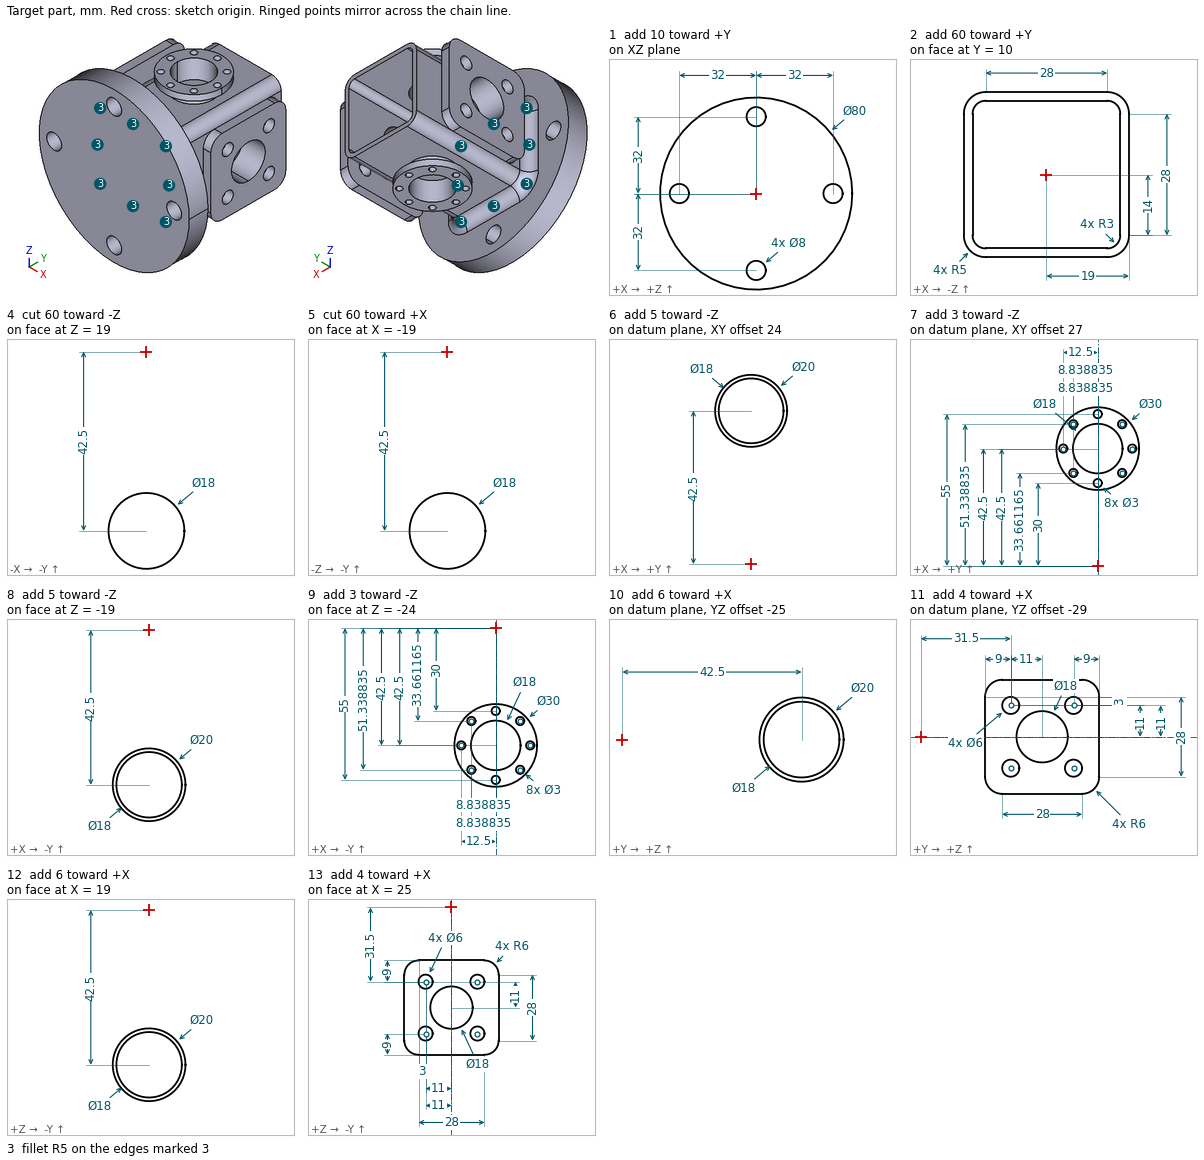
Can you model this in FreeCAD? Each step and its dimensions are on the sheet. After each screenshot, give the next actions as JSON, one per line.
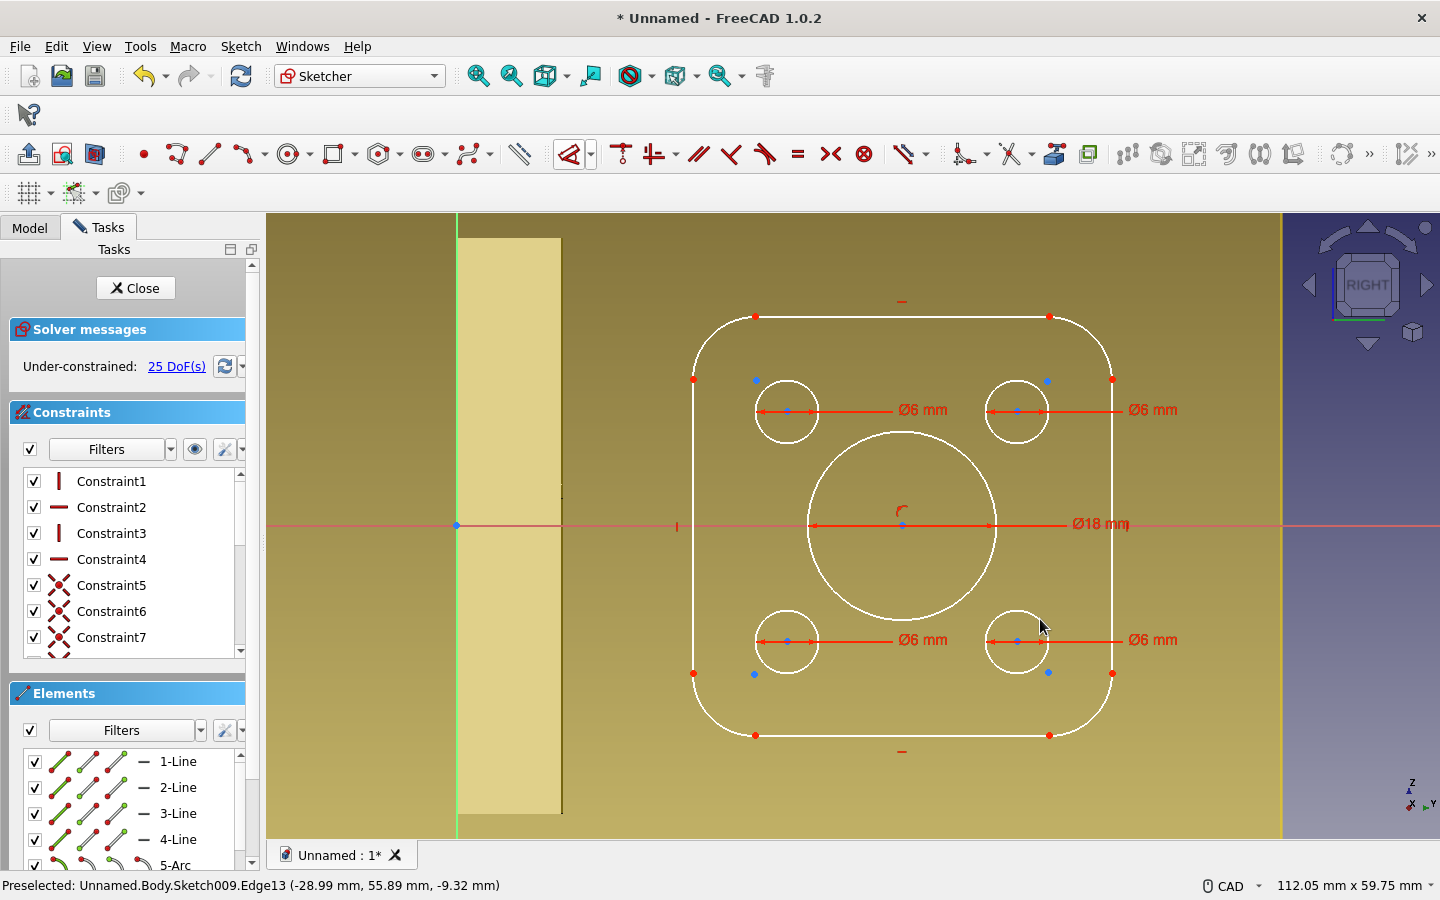
{"action": "left_click", "coordinate": [1112, 468]}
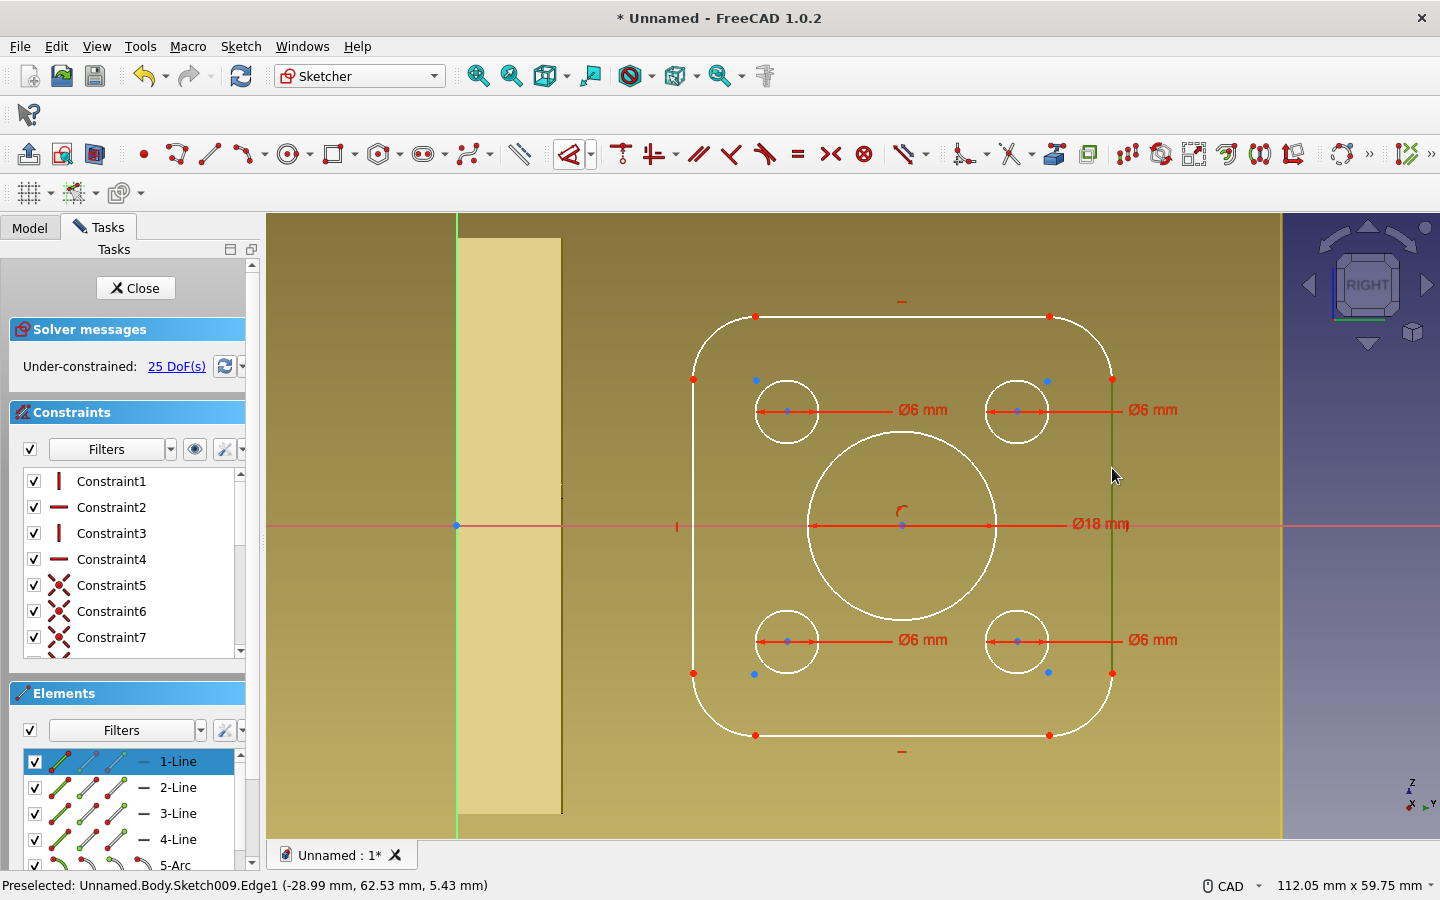
{"action": "left_click", "coordinate": [1077, 729]}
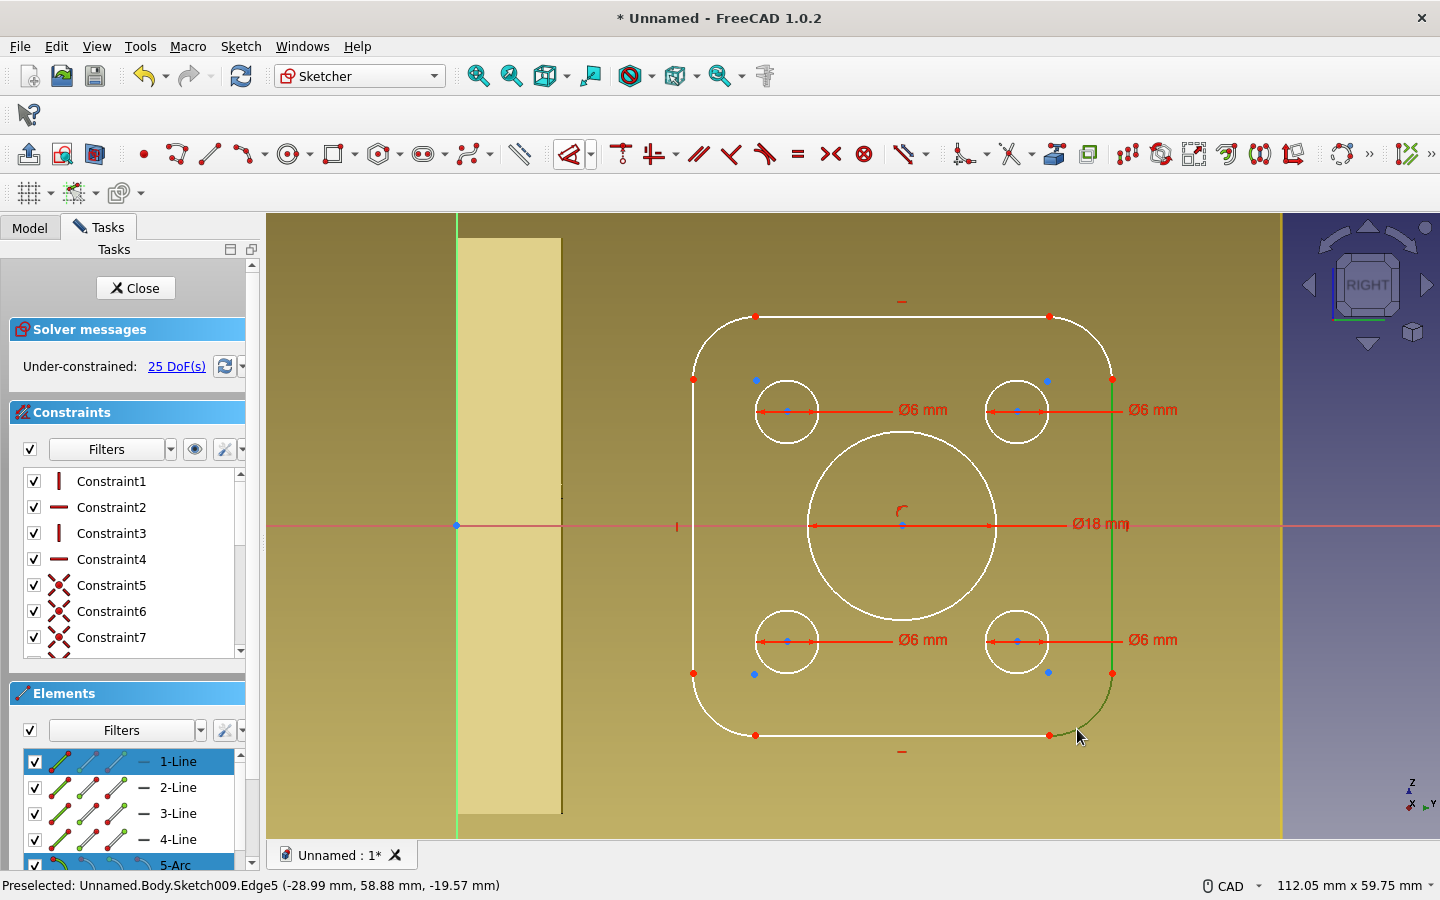
{"action": "key", "text": "t"}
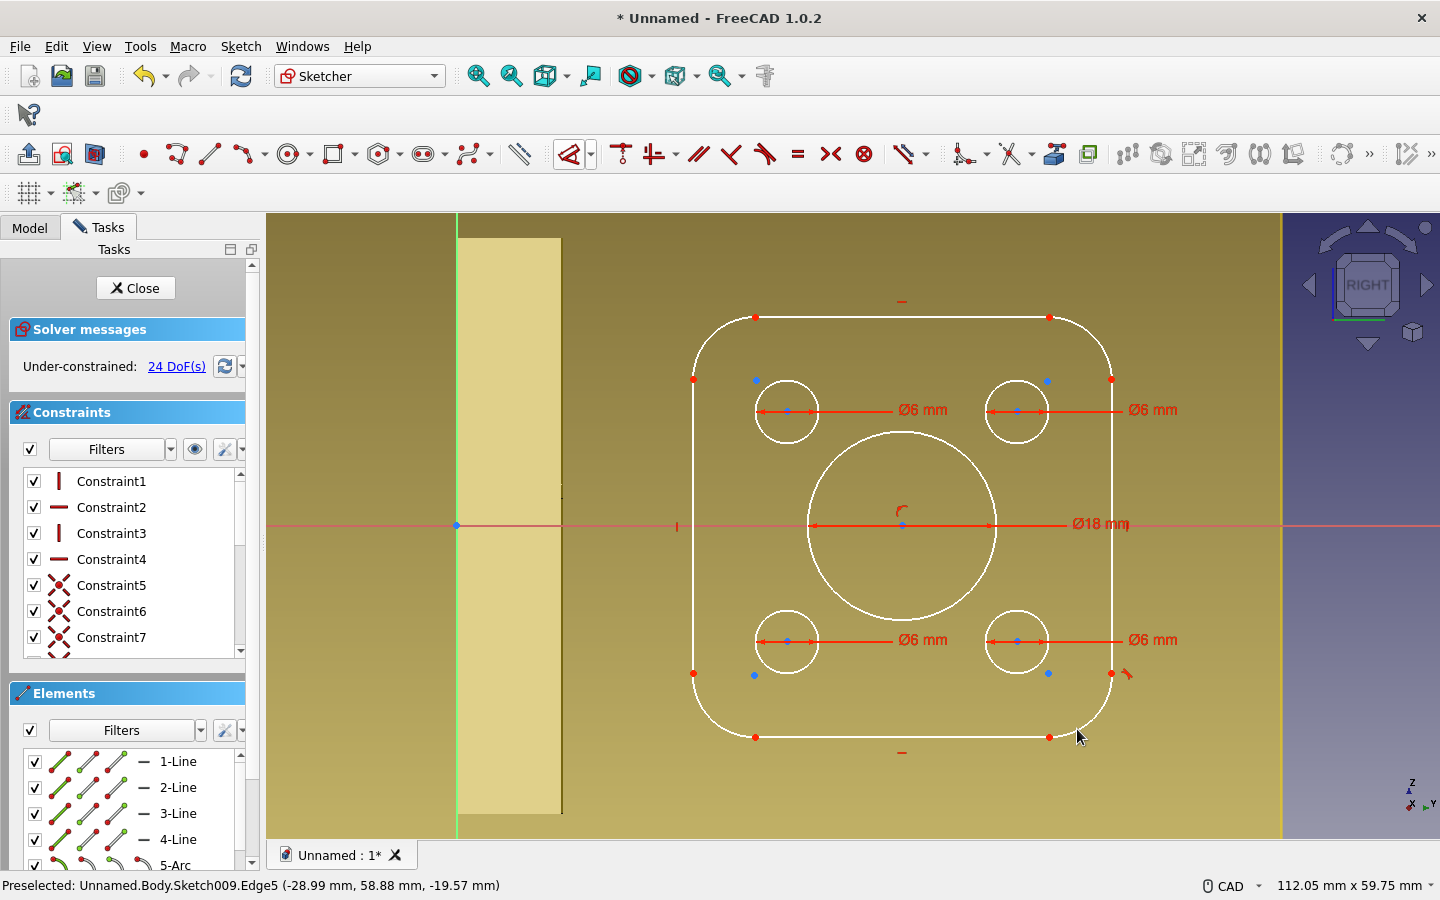
{"action": "left_click", "coordinate": [1112, 468]}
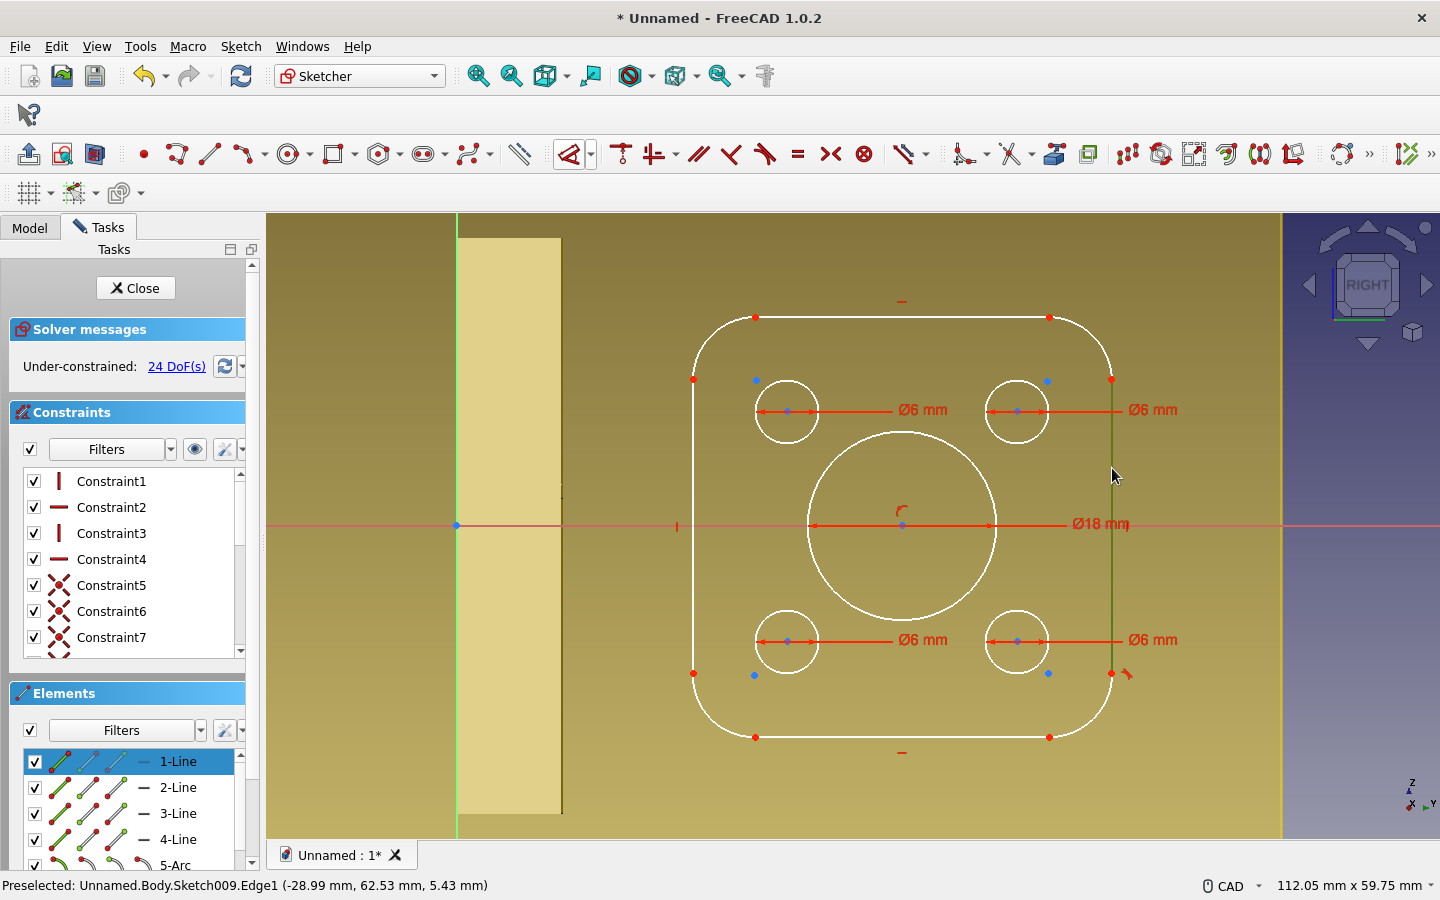
{"action": "left_click", "coordinate": [1105, 352]}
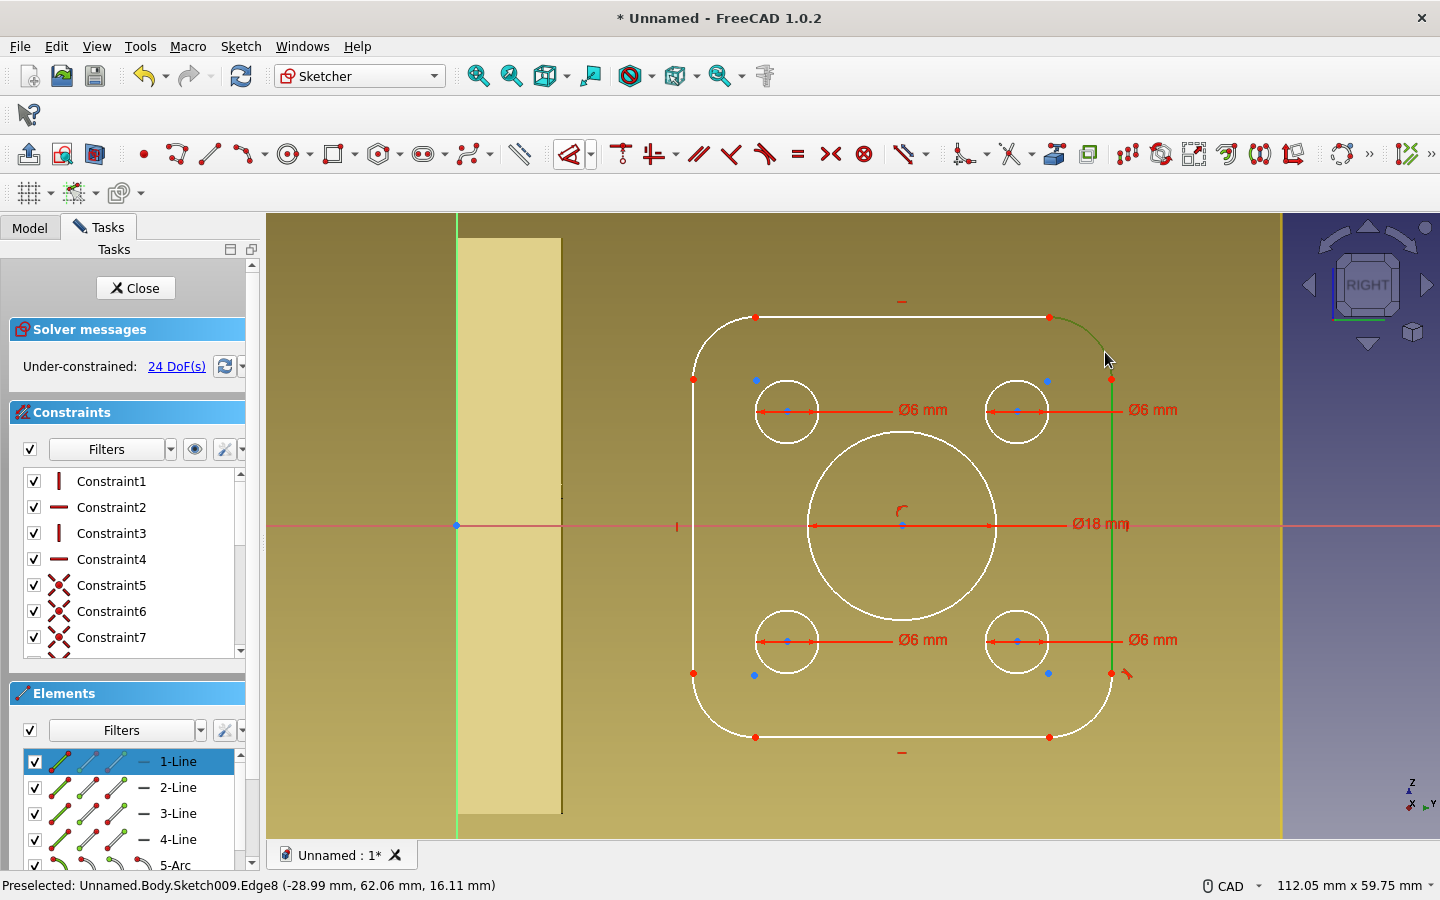
{"action": "key", "text": "t"}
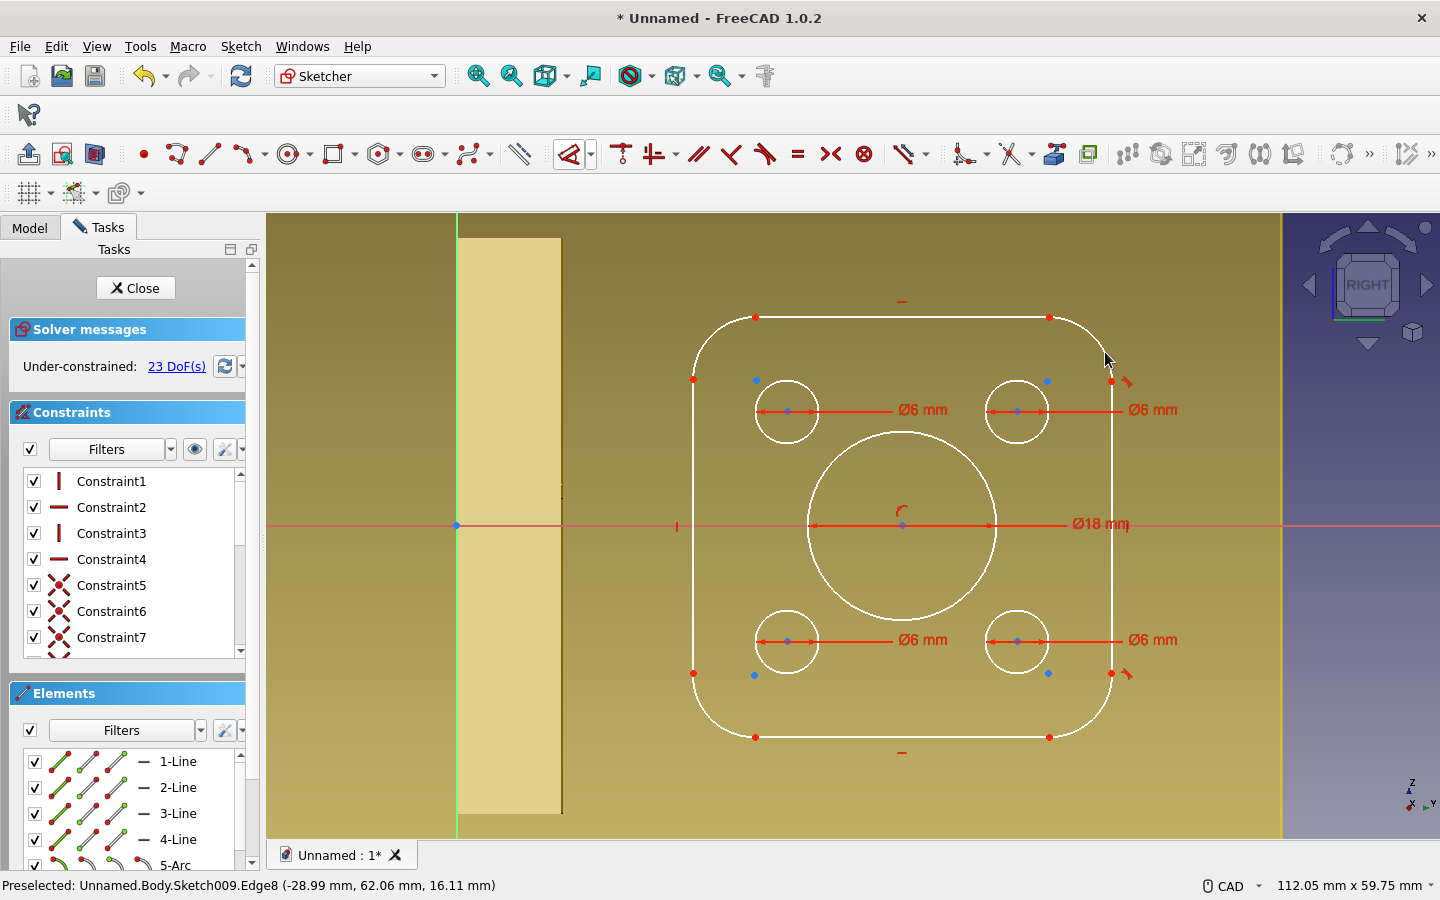
{"action": "left_click", "coordinate": [961, 737]}